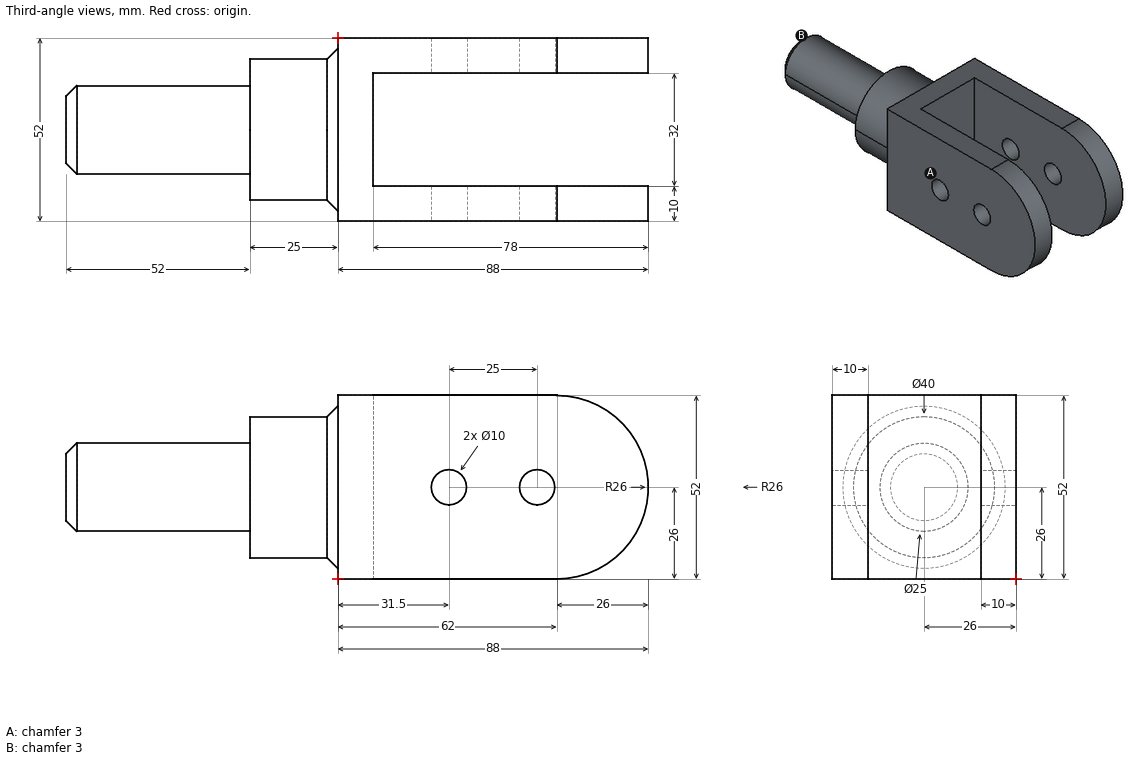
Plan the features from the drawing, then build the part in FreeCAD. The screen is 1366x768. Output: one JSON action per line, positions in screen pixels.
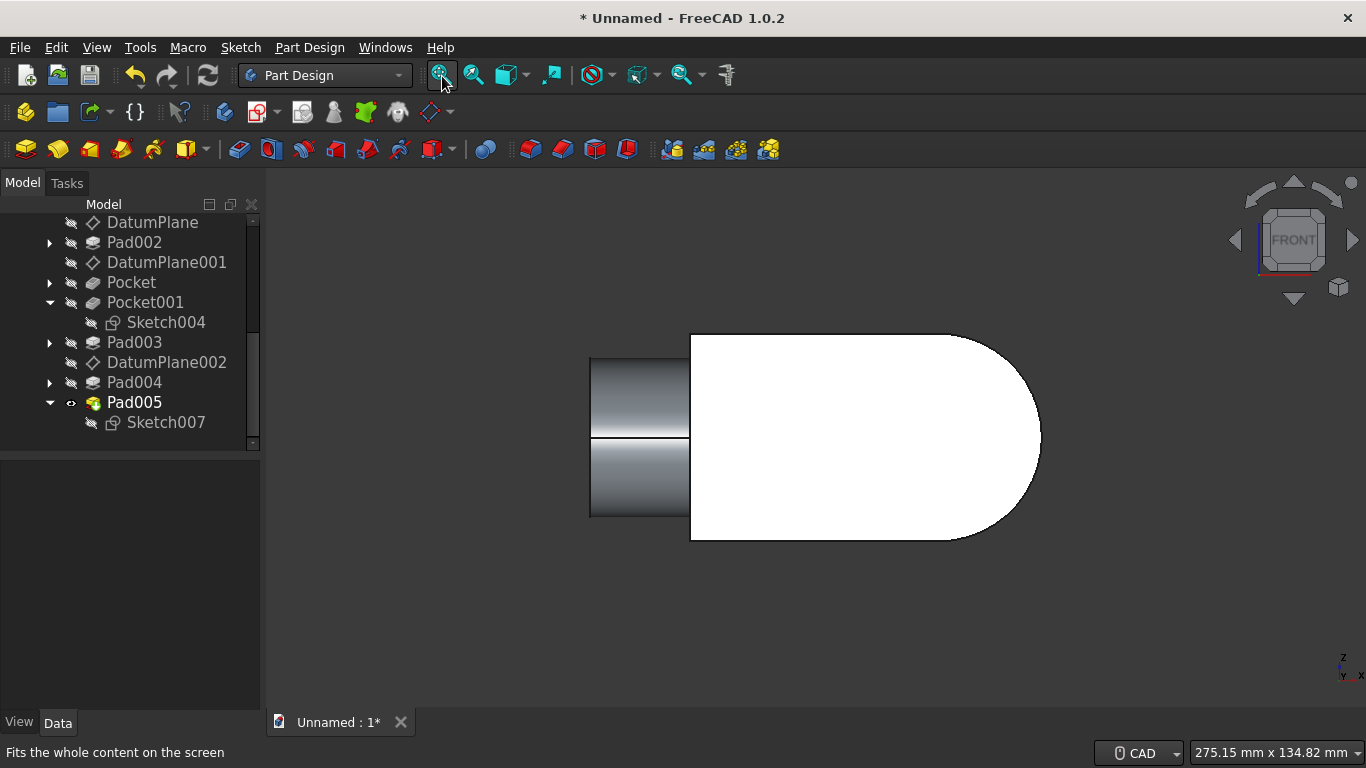
{"action": "left_click", "coordinate": [442, 76]}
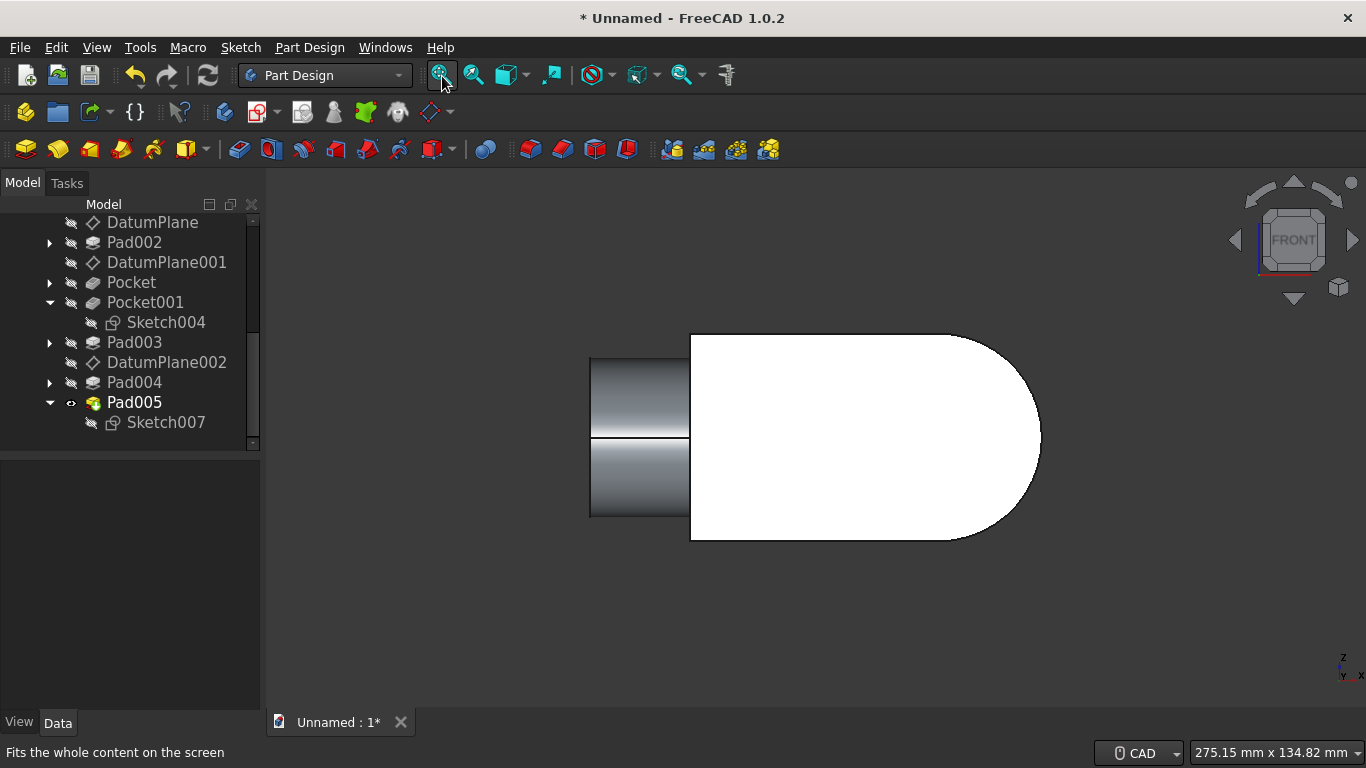
{"action": "key", "text": "3"}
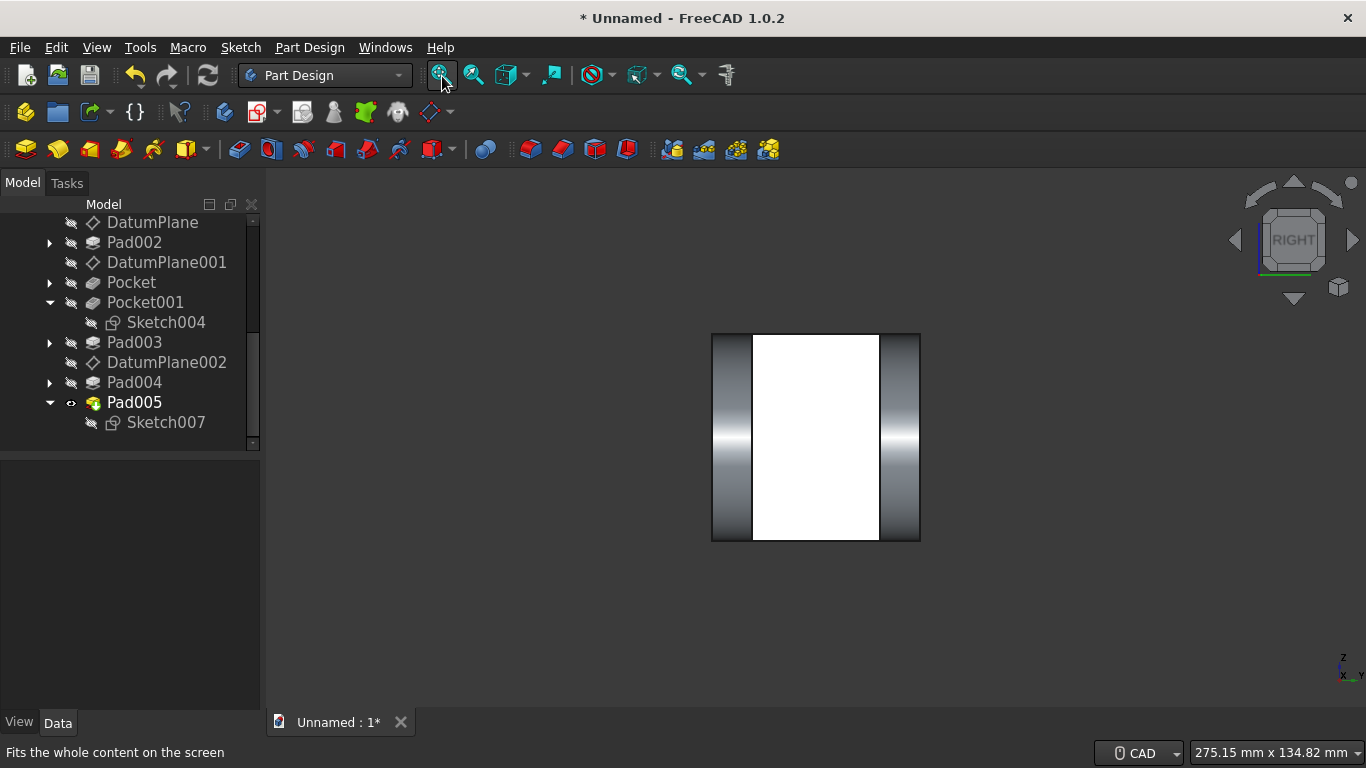
{"action": "left_click", "coordinate": [442, 76]}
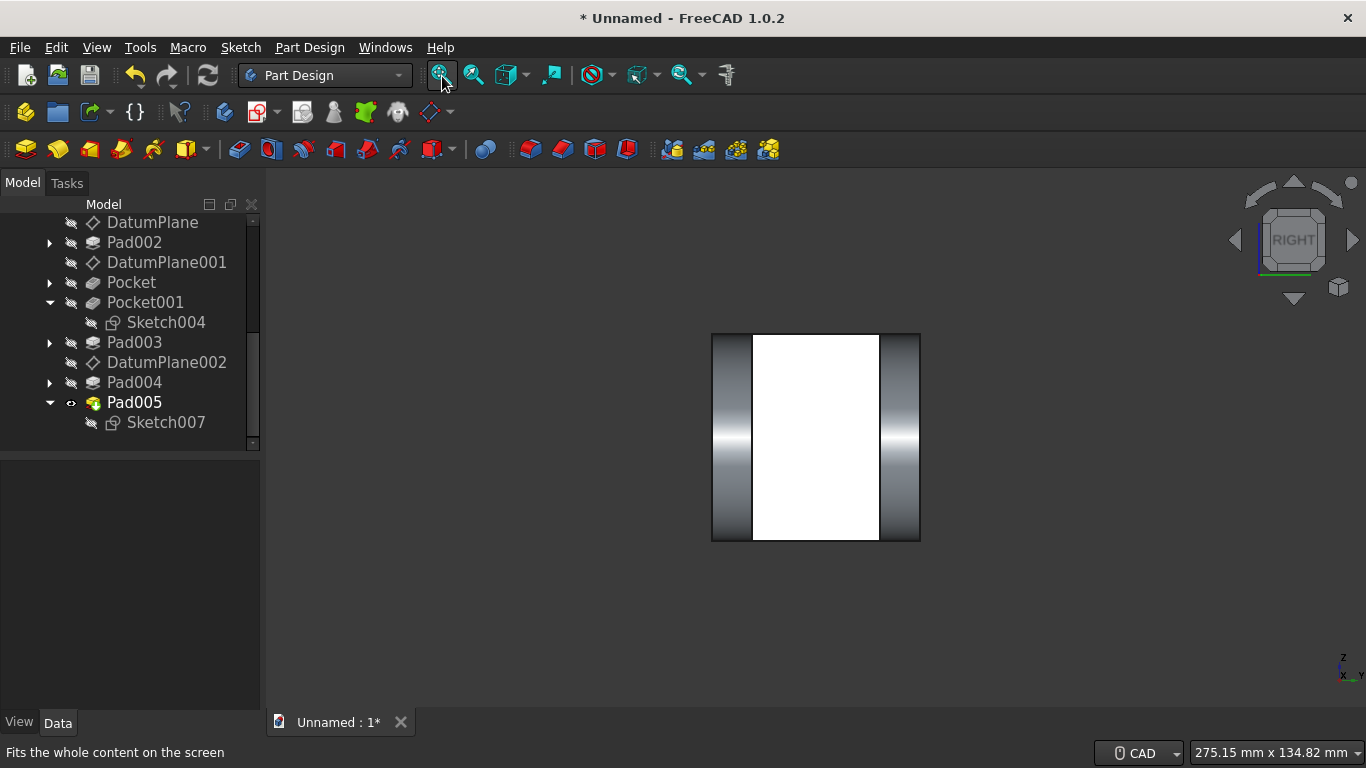
{"action": "key", "text": "5"}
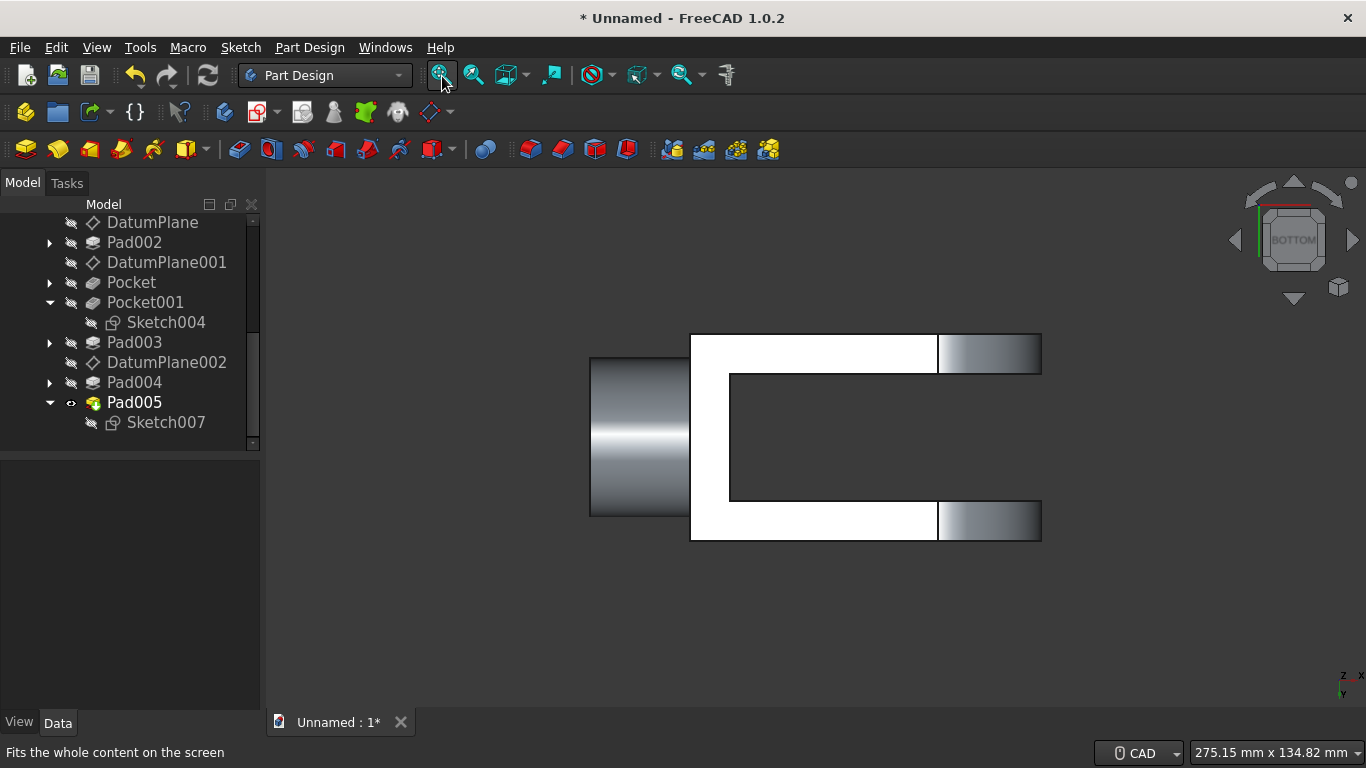
{"action": "left_click", "coordinate": [442, 76]}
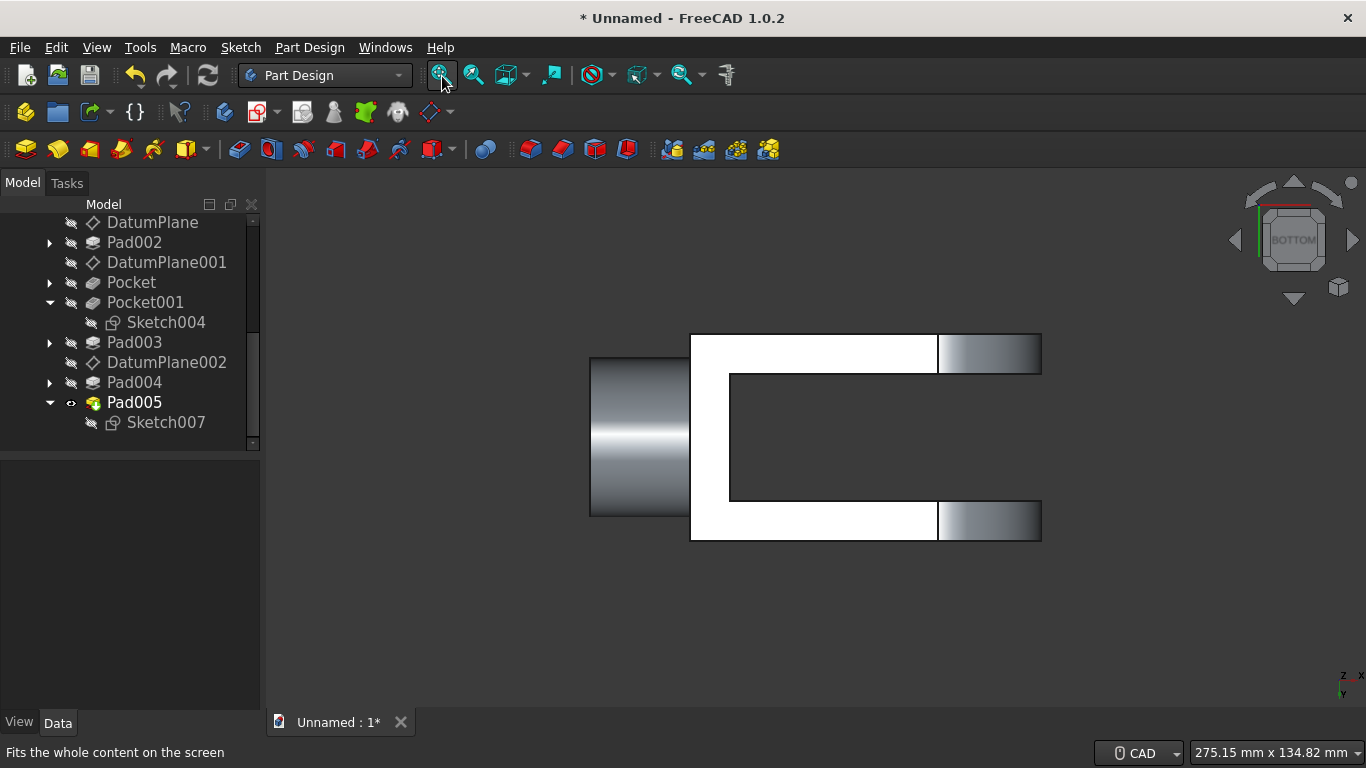
{"action": "key", "text": "4"}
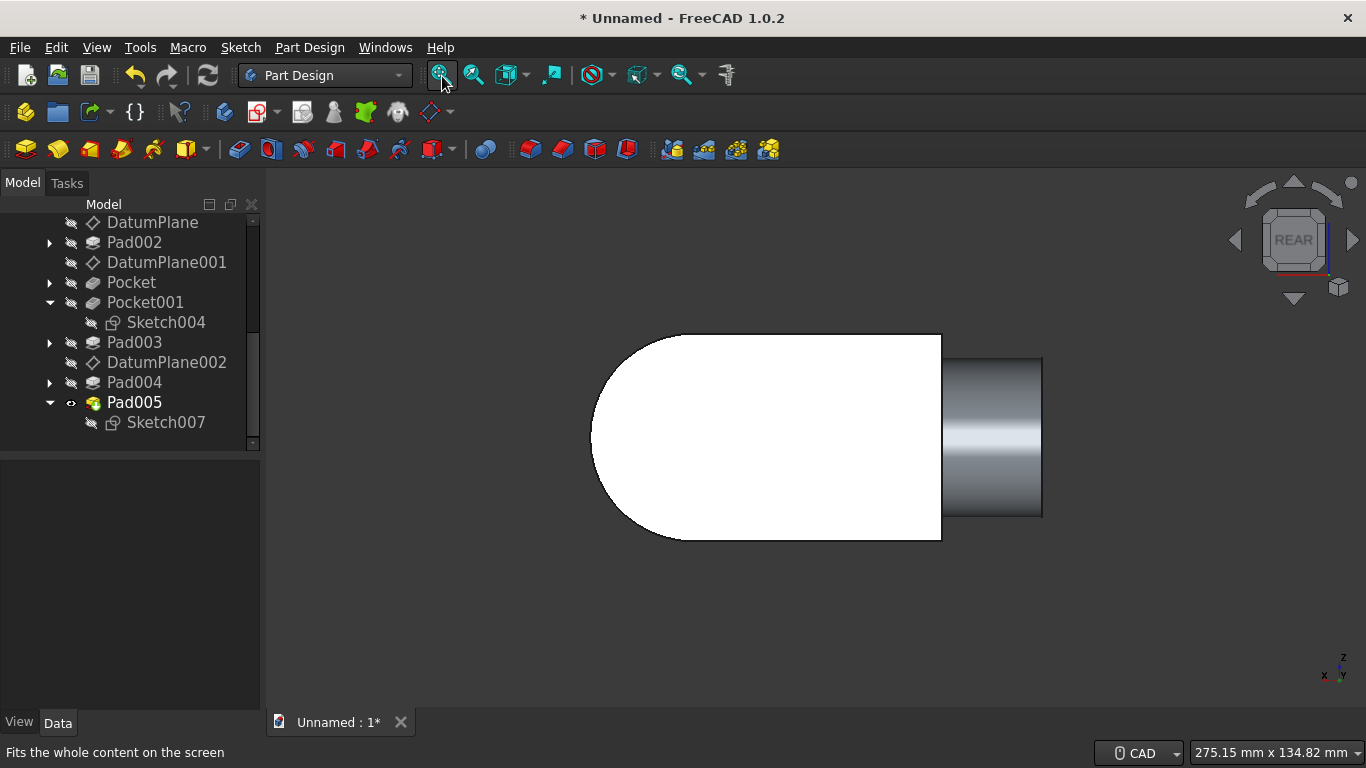
{"action": "left_click", "coordinate": [442, 76]}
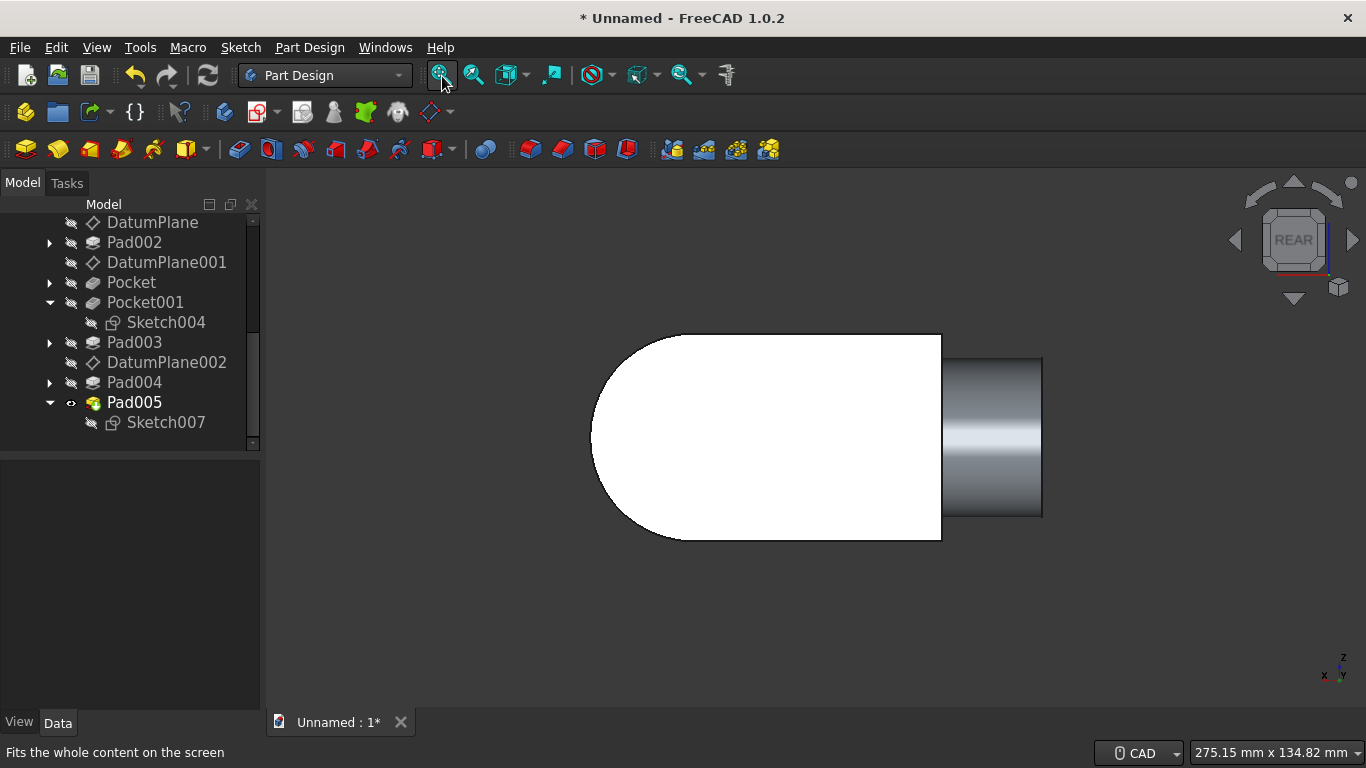
{"action": "key", "text": "6"}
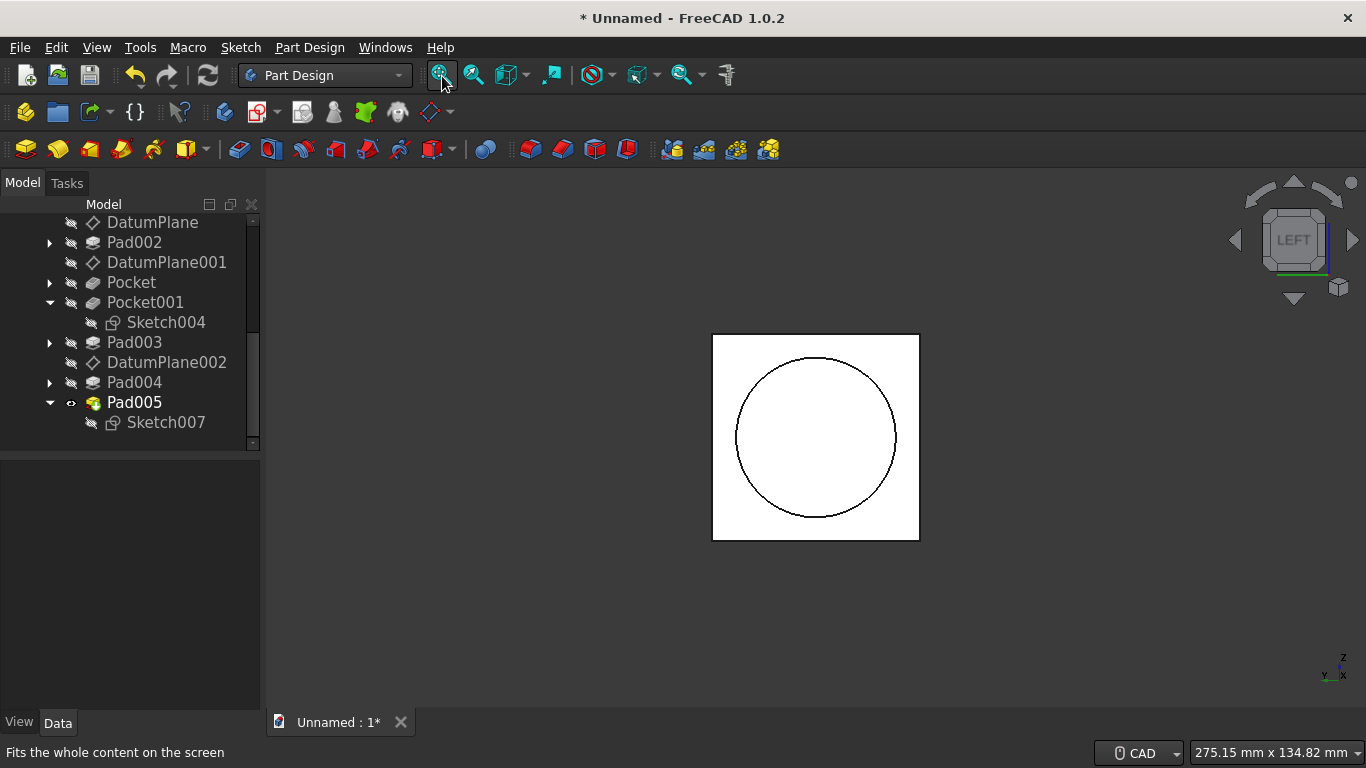
{"action": "left_click", "coordinate": [442, 76]}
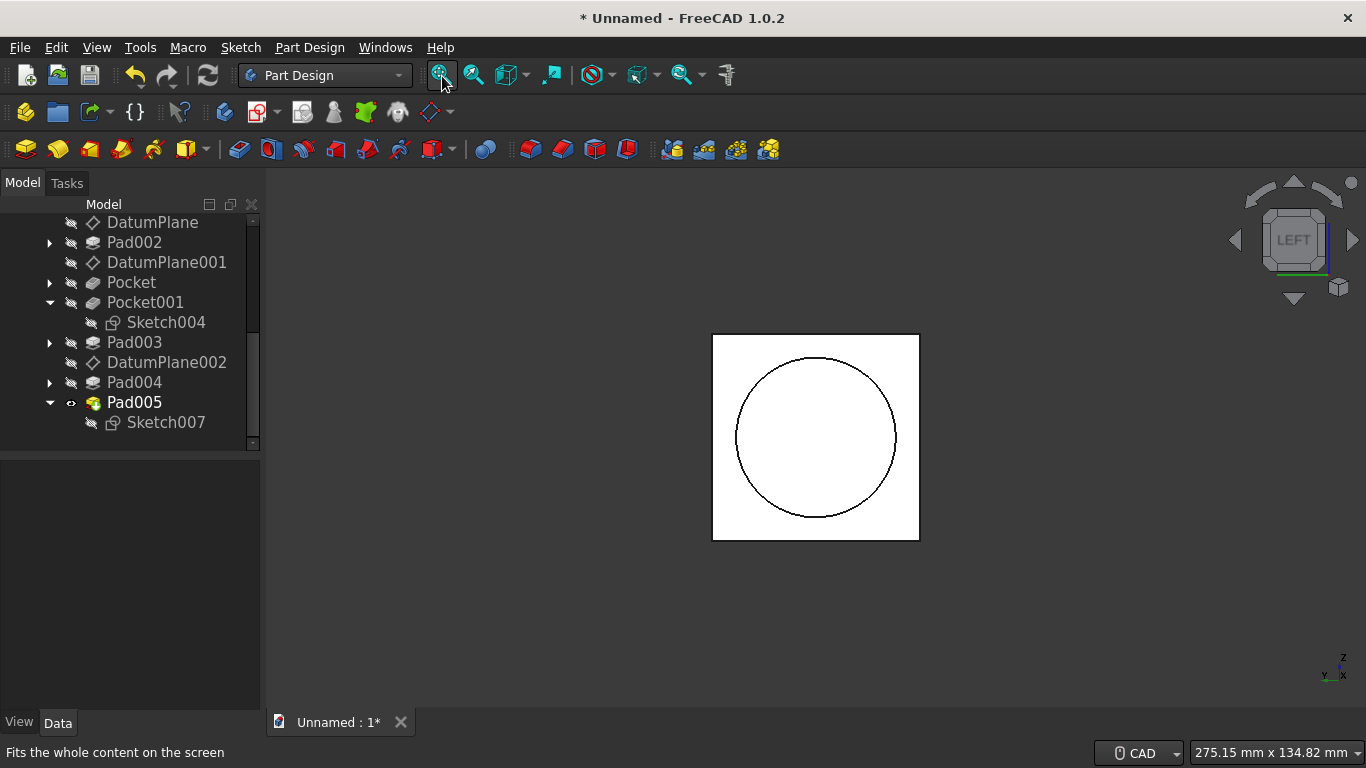
{"action": "key", "text": "v 3"}